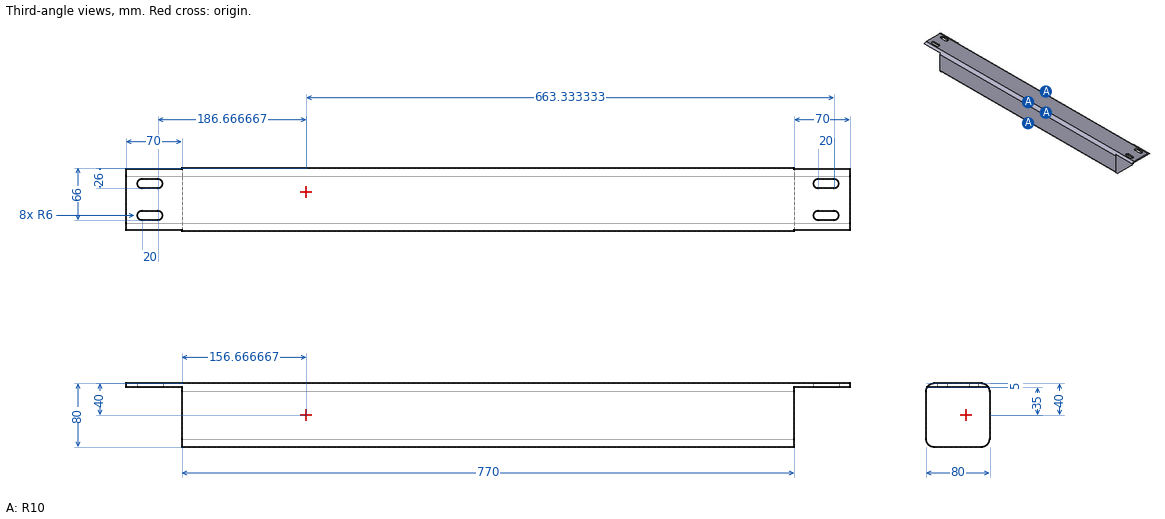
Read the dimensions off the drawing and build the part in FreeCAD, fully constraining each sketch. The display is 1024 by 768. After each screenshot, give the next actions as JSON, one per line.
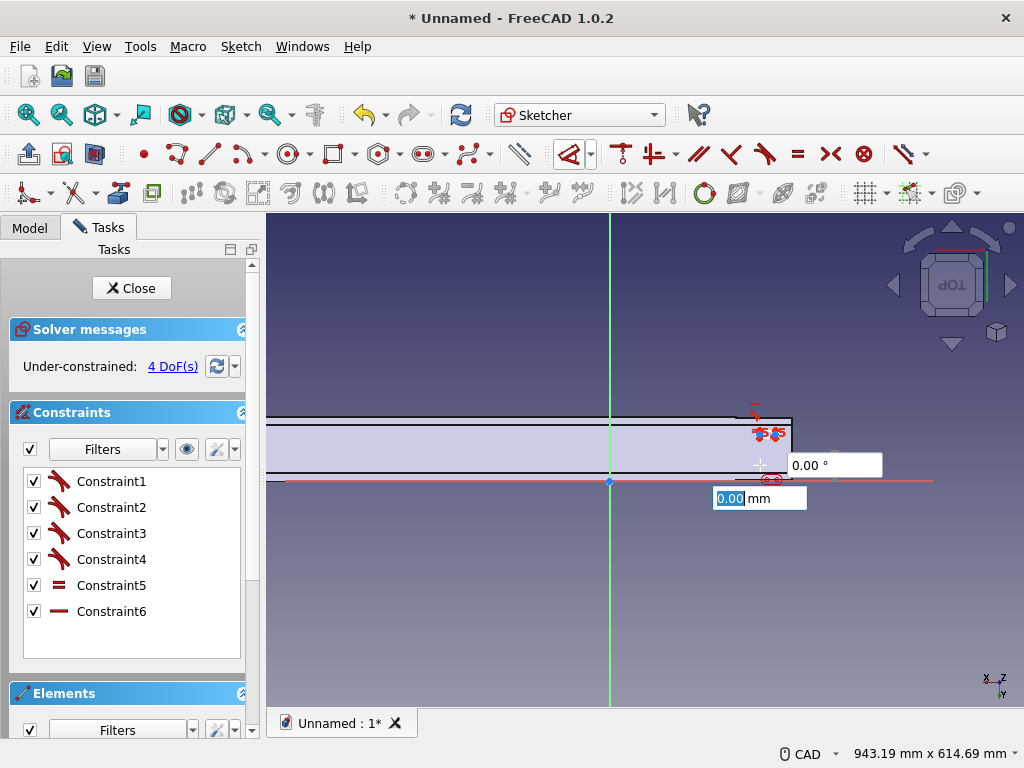
{"action": "left_click", "coordinate": [776, 465]}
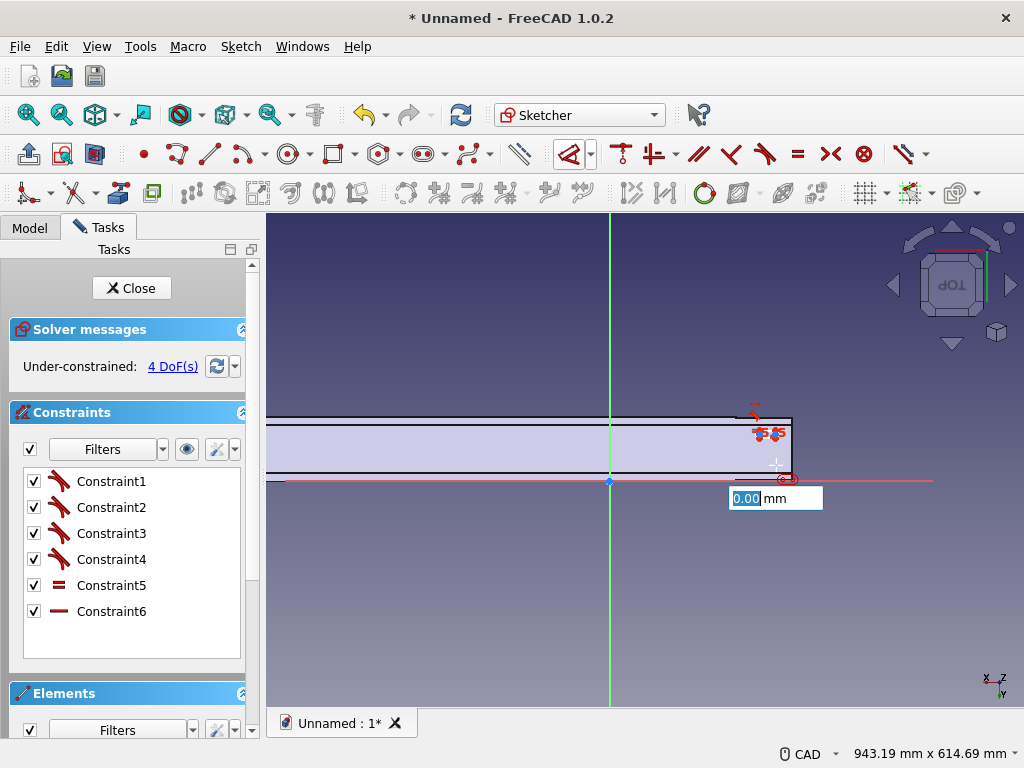
{"action": "scroll", "coordinate": [768, 461], "scroll_direction": "up", "scroll_amount": 6}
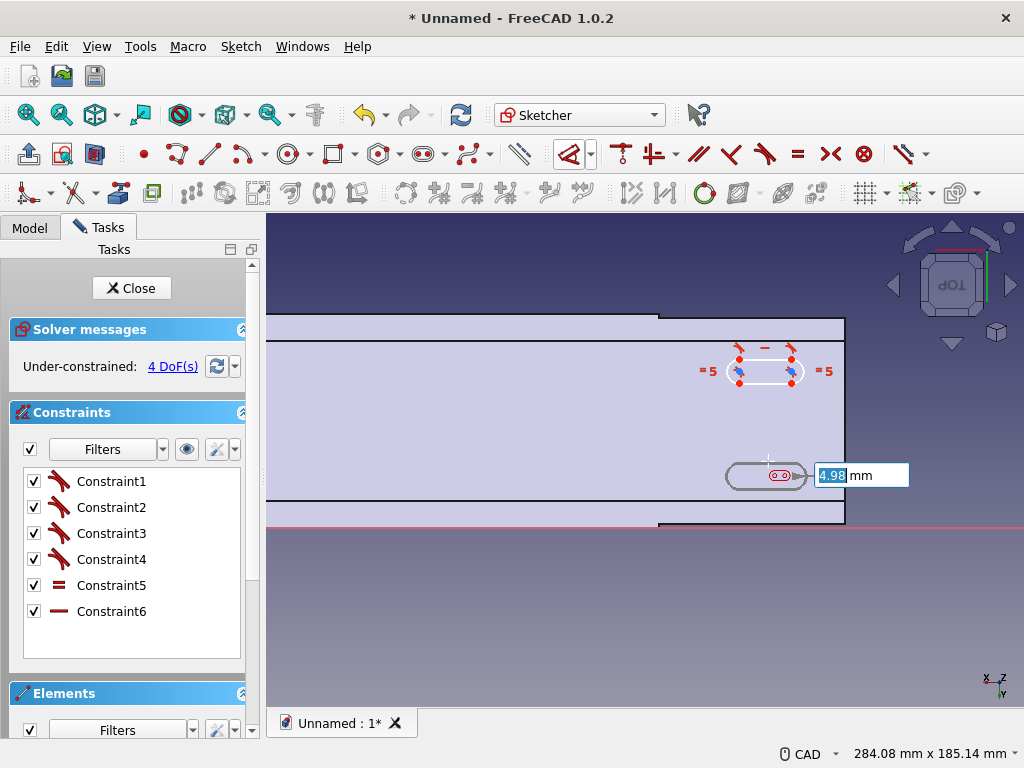
{"action": "left_click", "coordinate": [765, 458]}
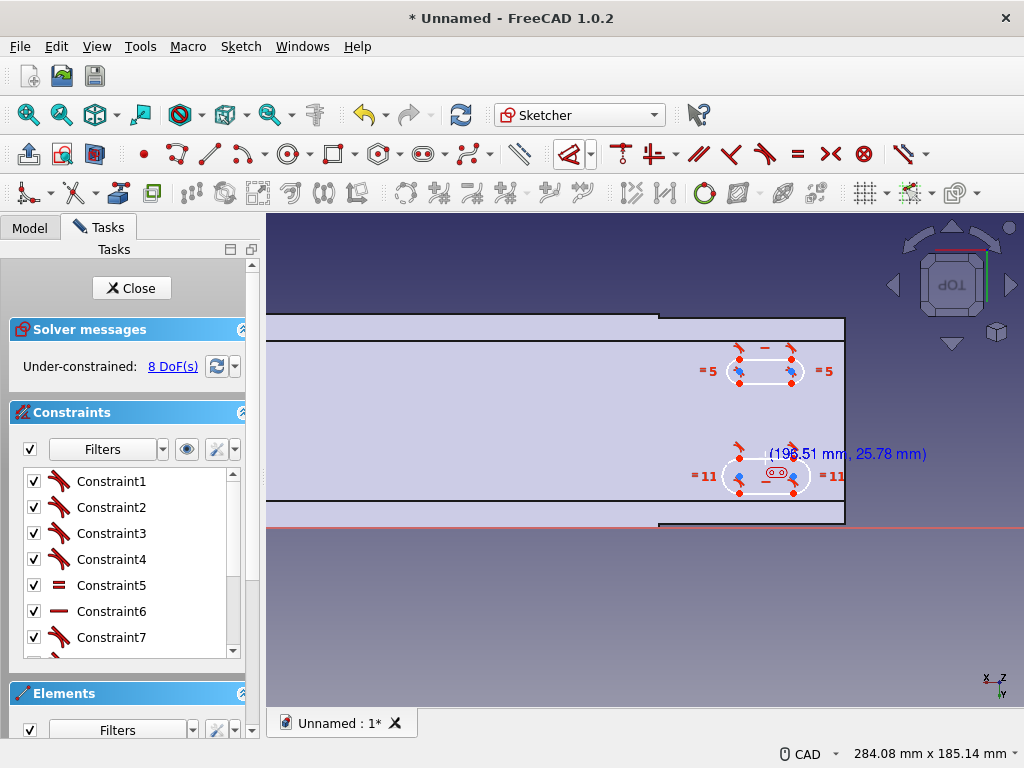
{"action": "scroll", "coordinate": [764, 464], "scroll_direction": "down", "scroll_amount": 9}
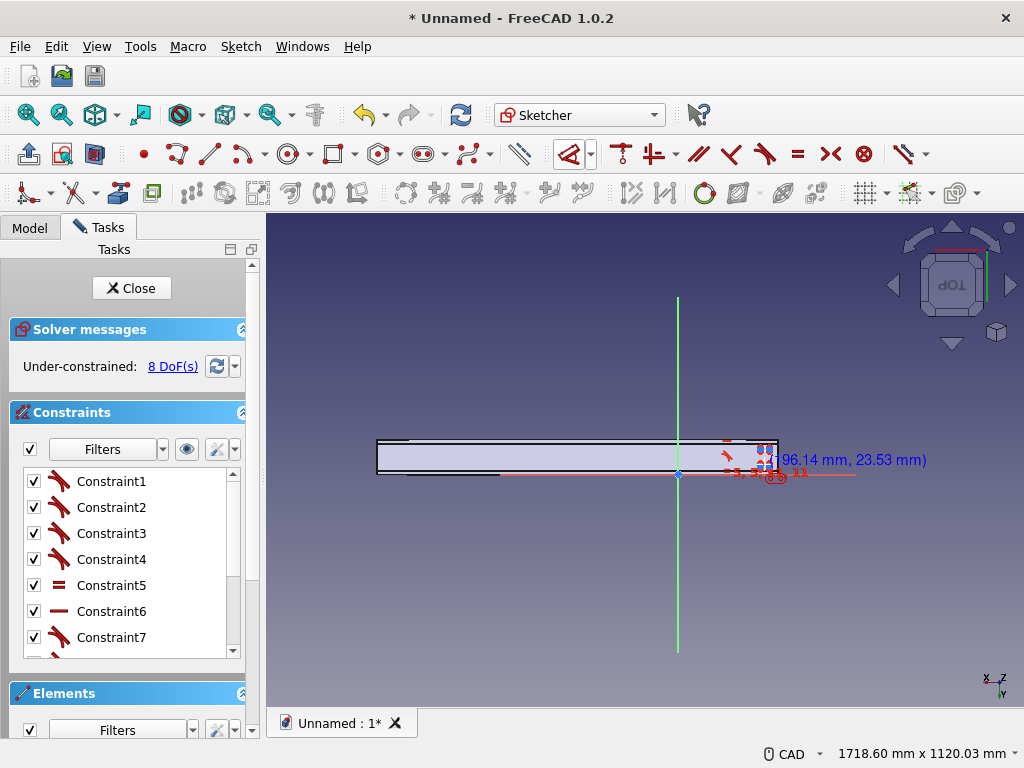
{"action": "scroll", "coordinate": [385, 466], "scroll_direction": "up", "scroll_amount": 11}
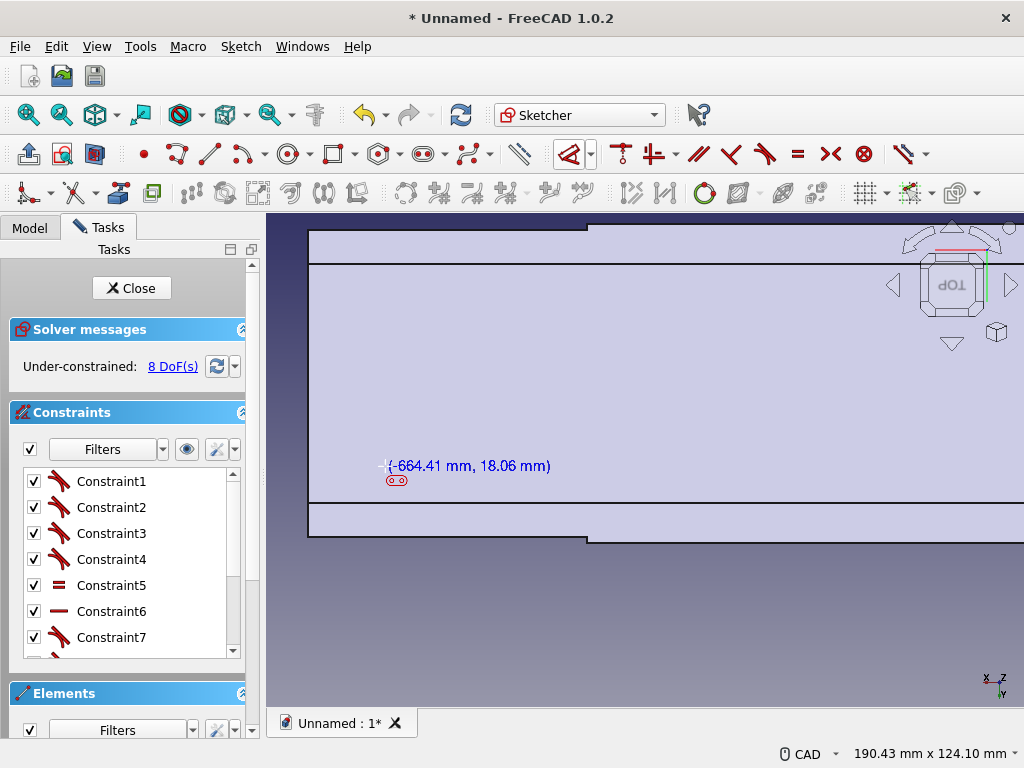
{"action": "scroll", "coordinate": [384, 466], "scroll_direction": "down", "scroll_amount": 11}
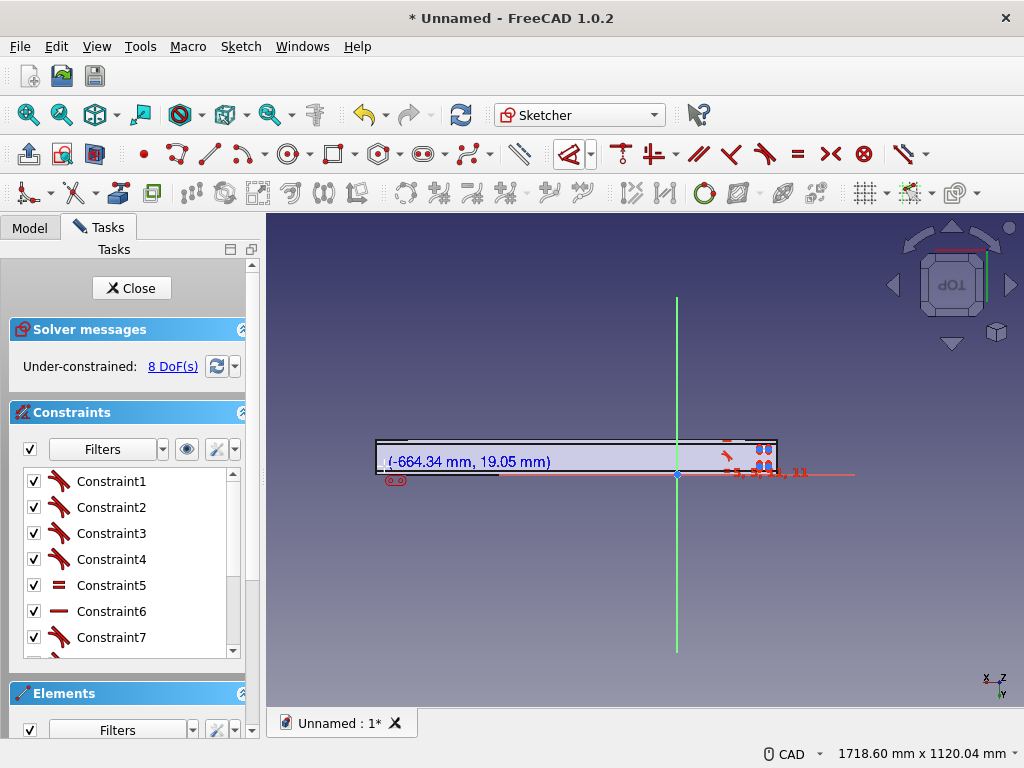
{"action": "scroll", "coordinate": [385, 466], "scroll_direction": "up", "scroll_amount": 3}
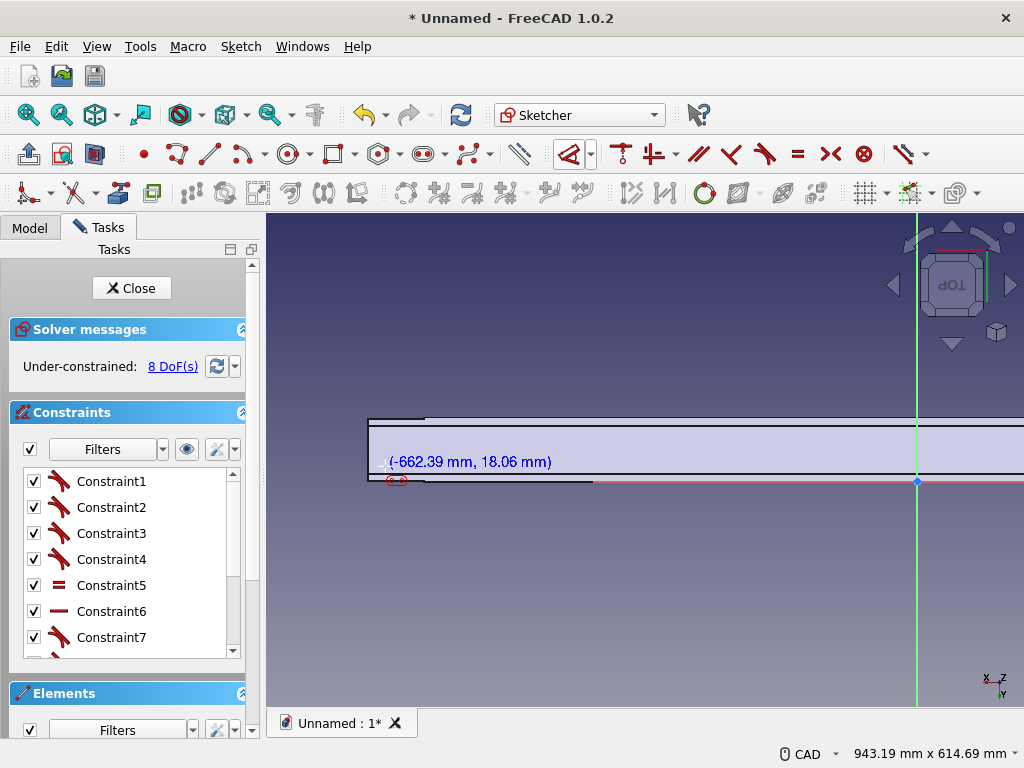
{"action": "left_click", "coordinate": [384, 466]}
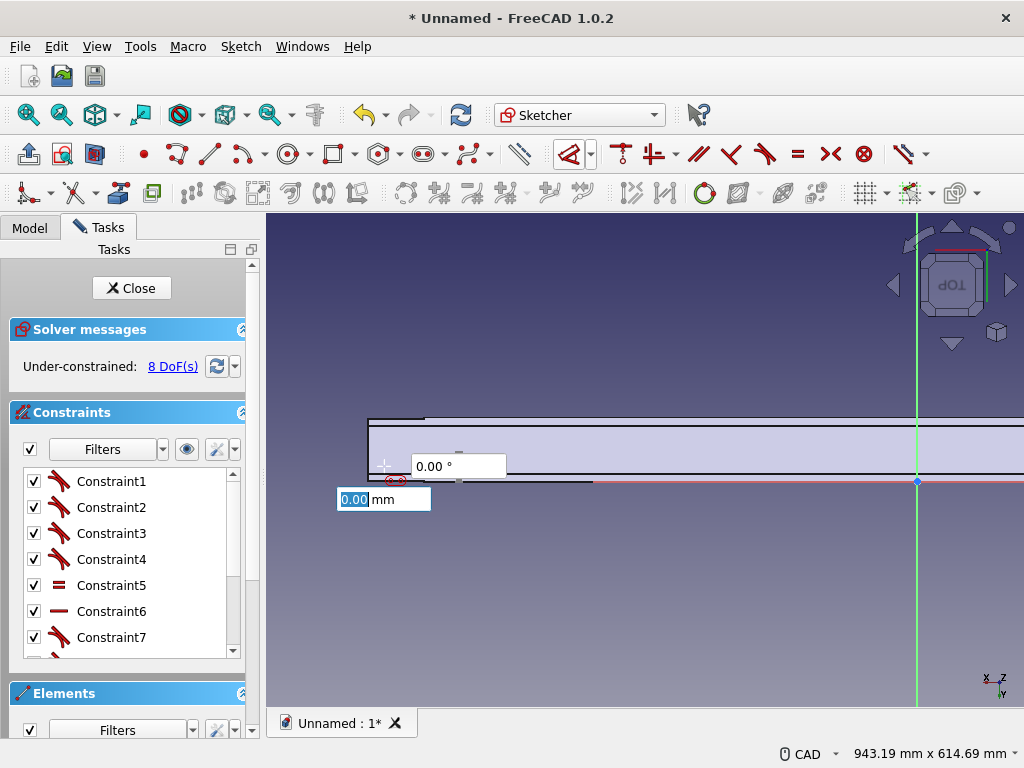
{"action": "left_click", "coordinate": [400, 466]}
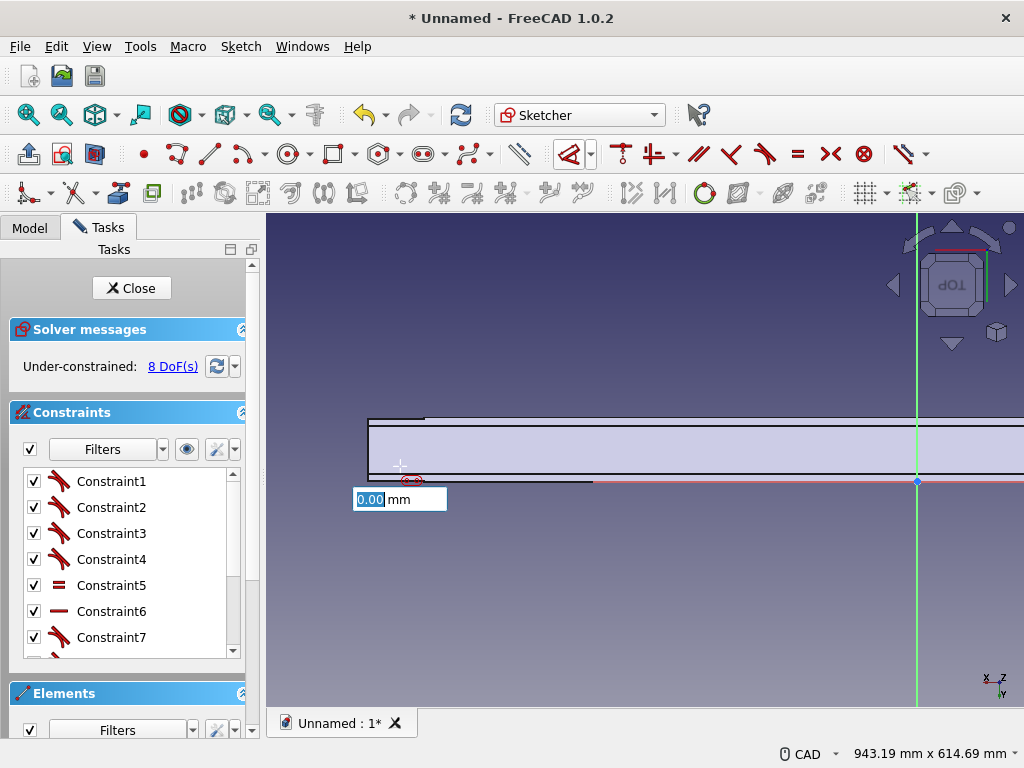
{"action": "scroll", "coordinate": [392, 461], "scroll_direction": "up", "scroll_amount": 6}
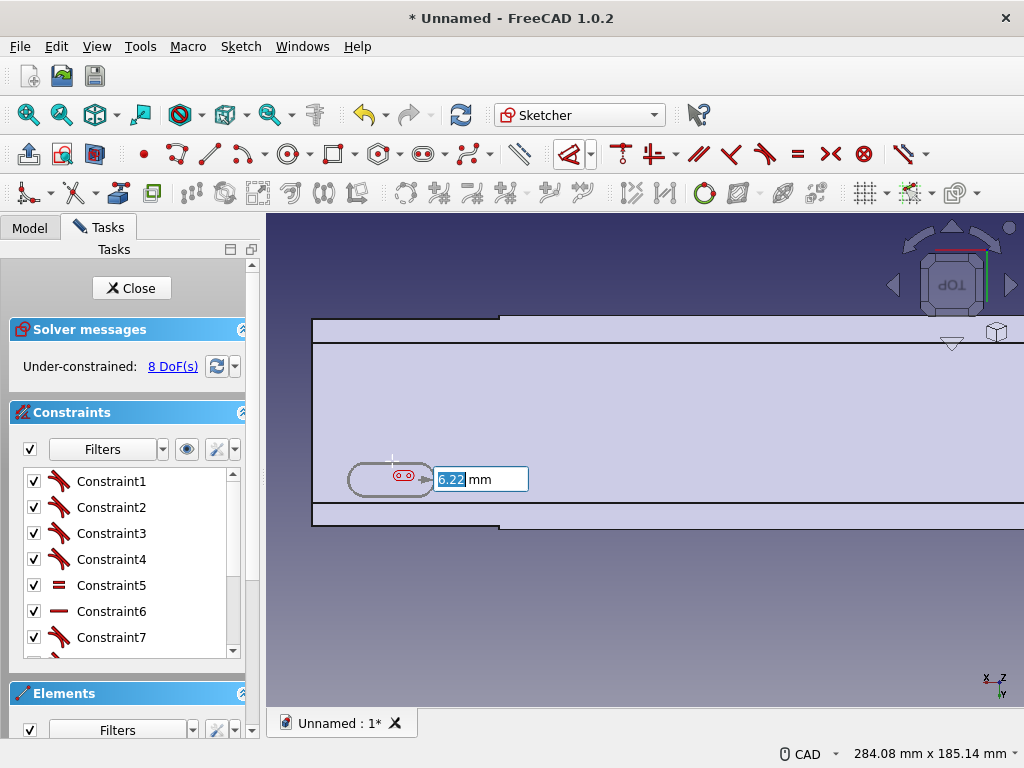
{"action": "left_click", "coordinate": [392, 460]}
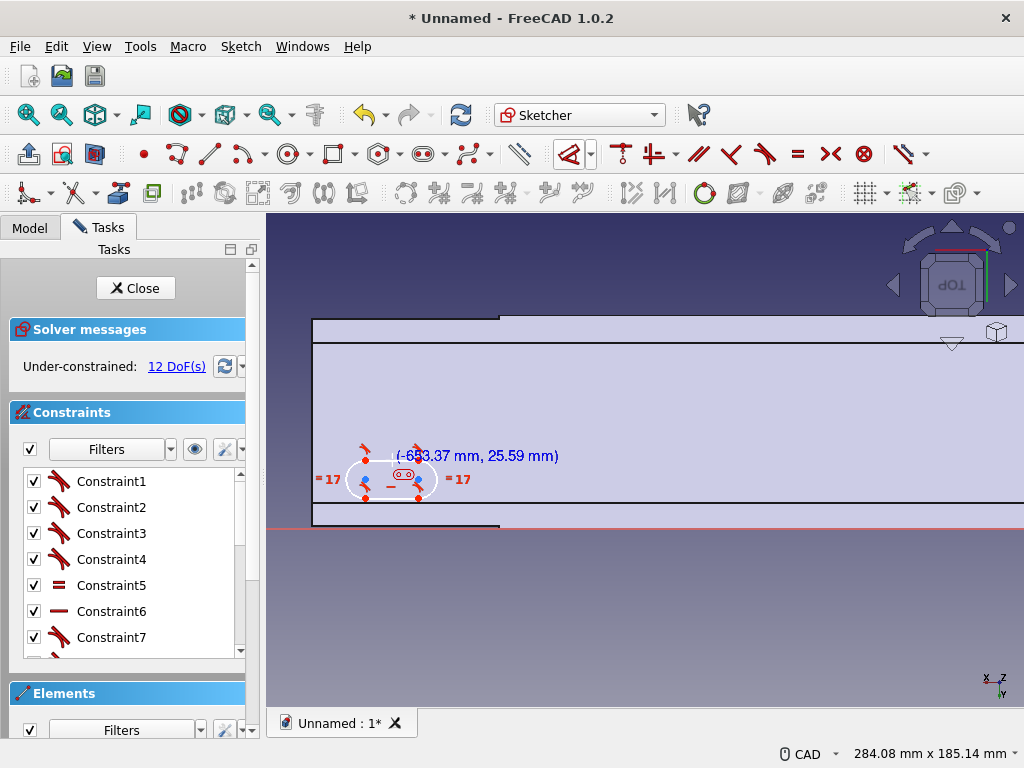
{"action": "scroll", "coordinate": [365, 369], "scroll_direction": "up", "scroll_amount": 2}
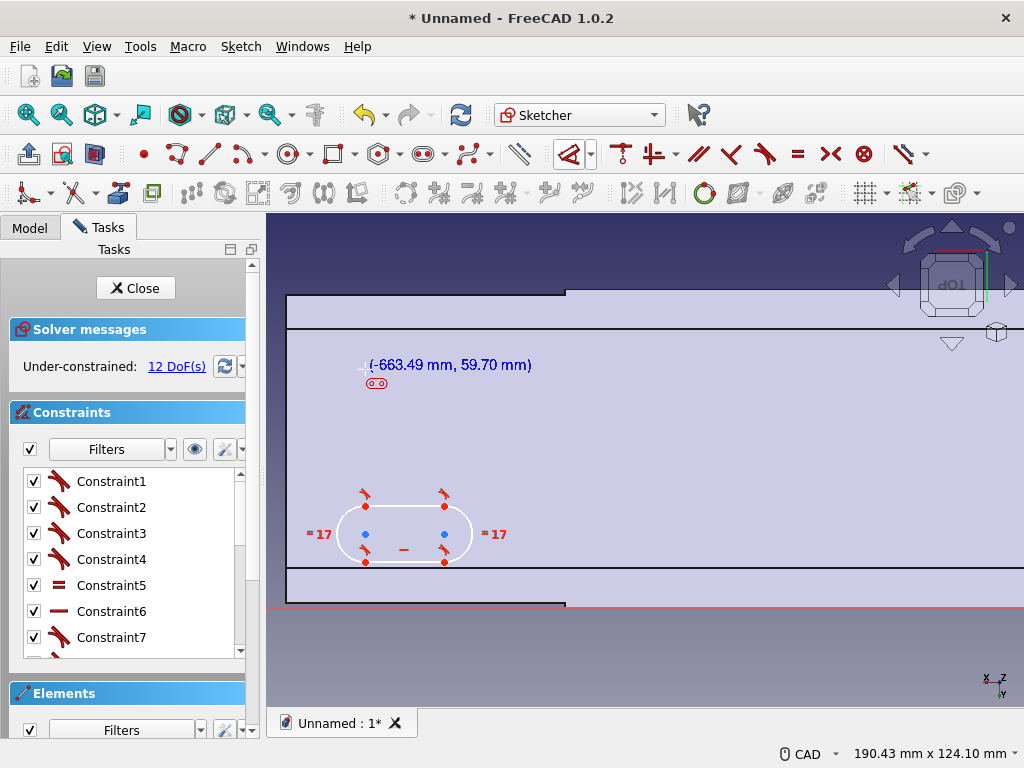
{"action": "scroll", "coordinate": [387, 458], "scroll_direction": "down", "scroll_amount": 11}